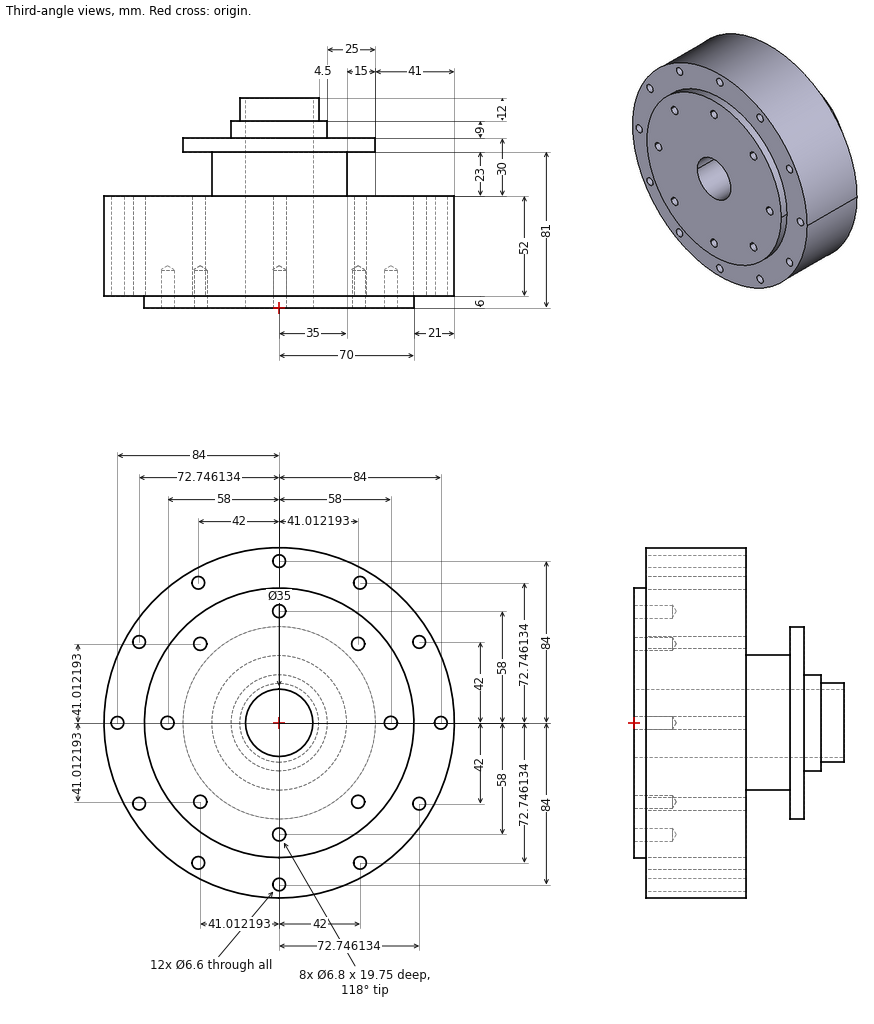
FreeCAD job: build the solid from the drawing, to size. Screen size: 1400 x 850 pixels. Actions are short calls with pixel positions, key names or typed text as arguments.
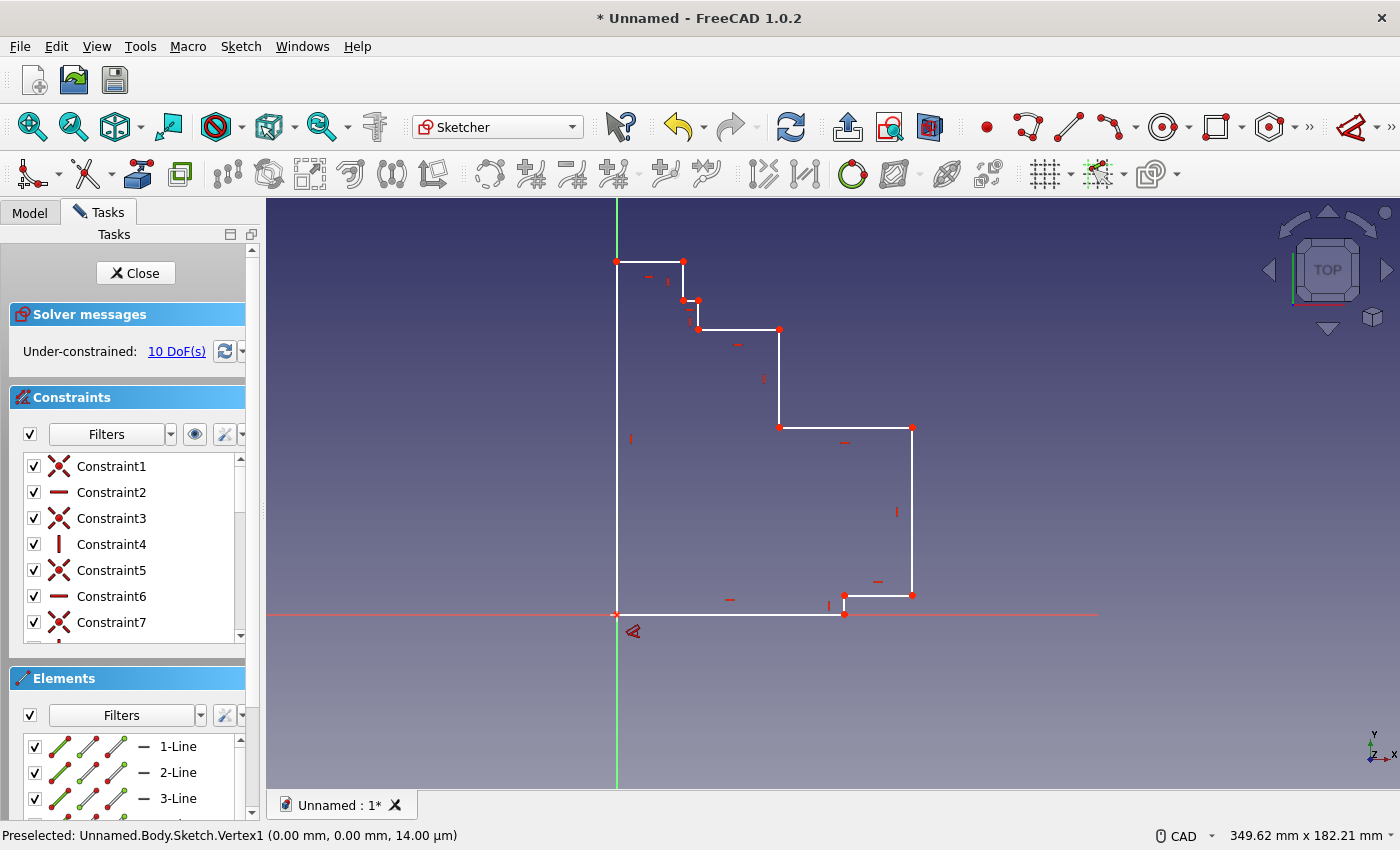
scroll(844, 605, up, 4)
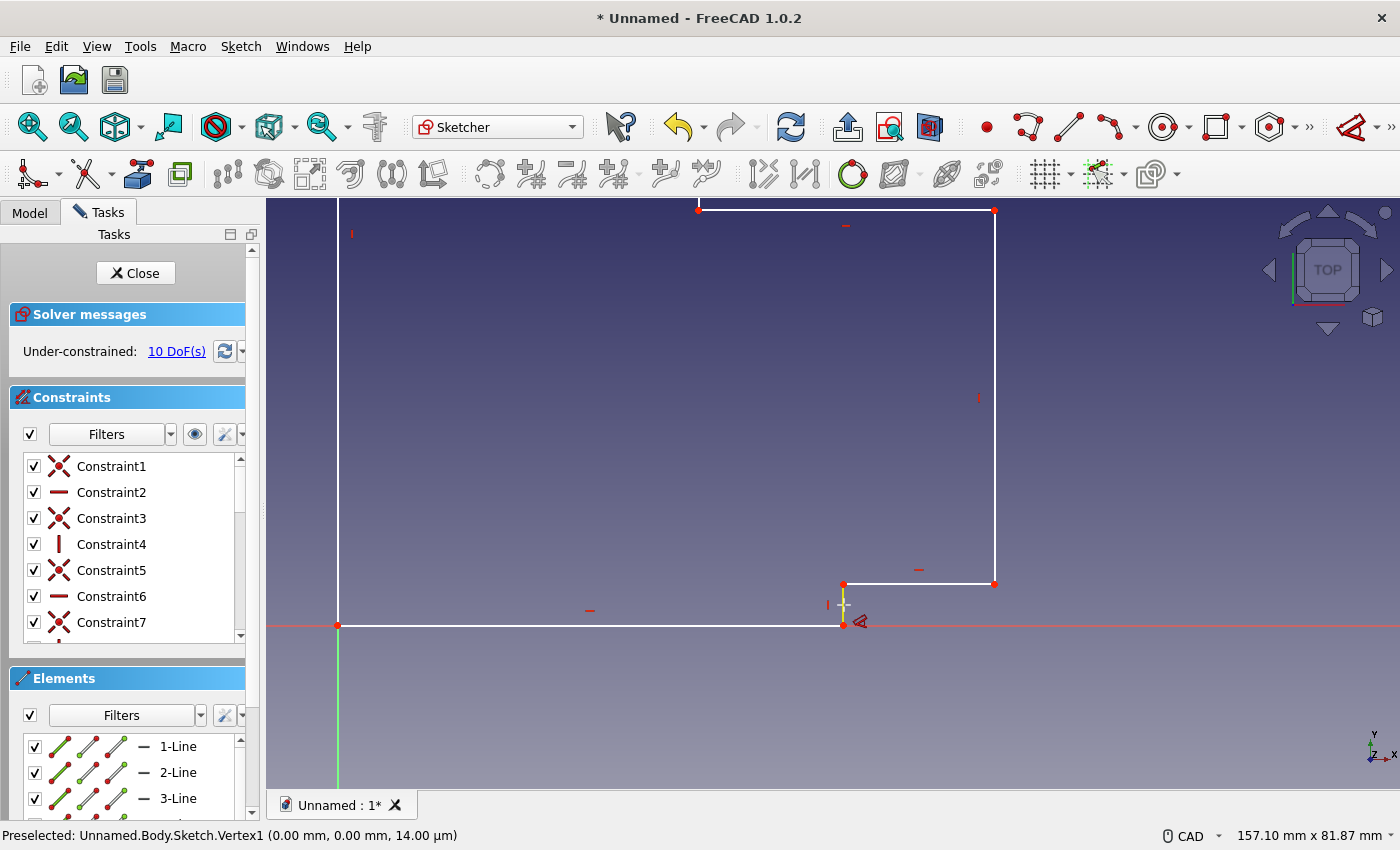
click(843, 605)
click(877, 605)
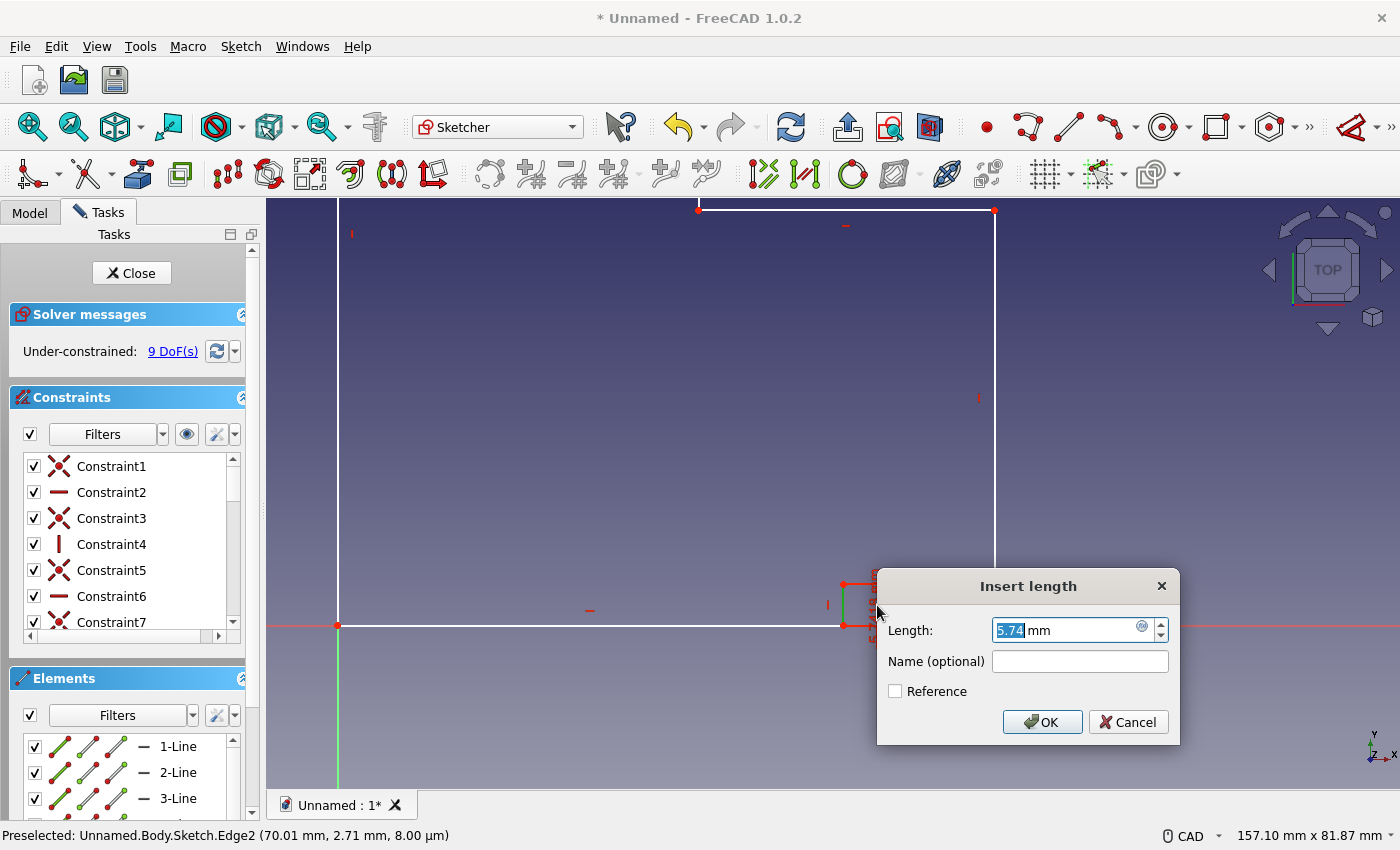
text(6)
key(Return)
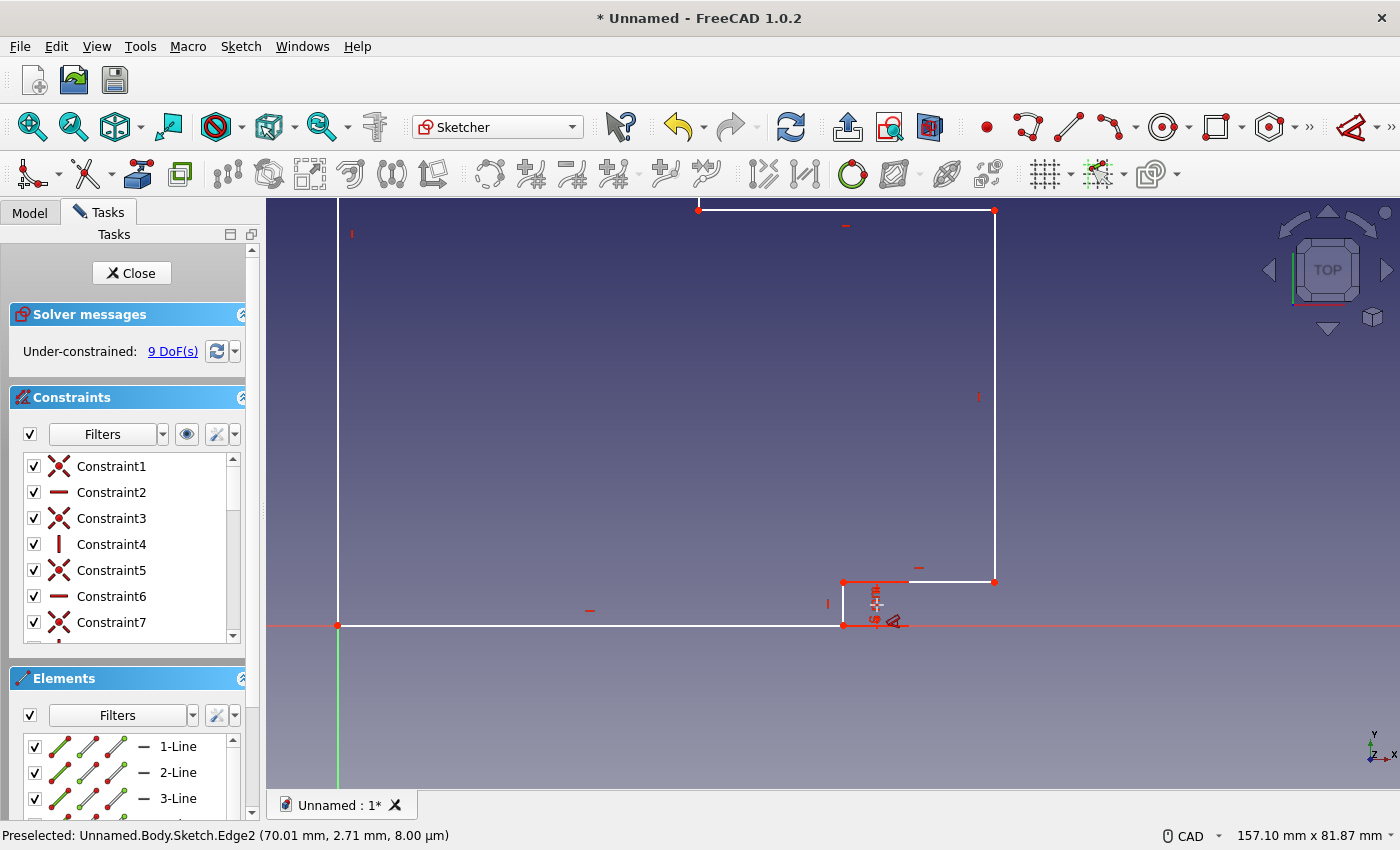
scroll(845, 707, down, 4)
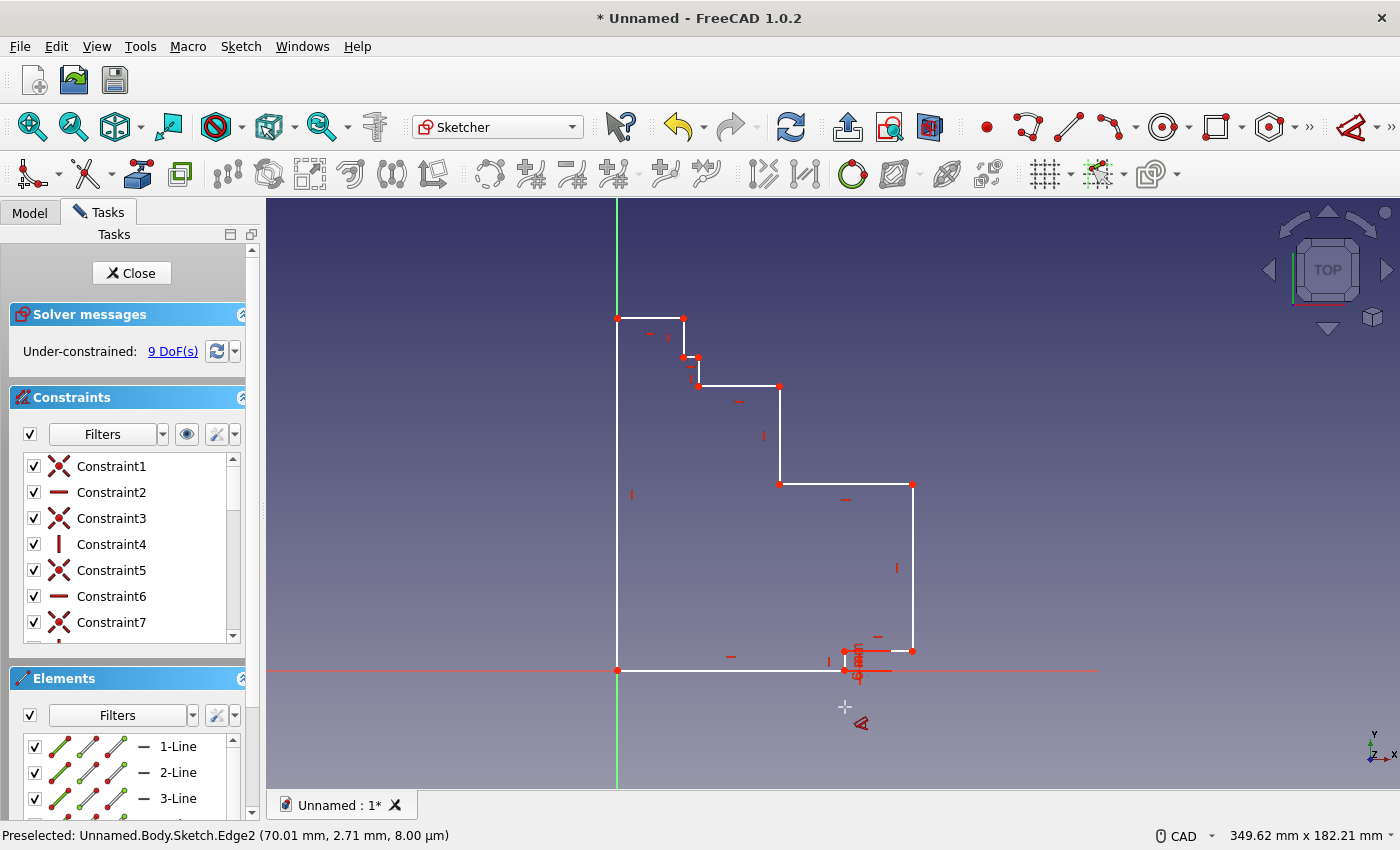
scroll(699, 378, up, 3)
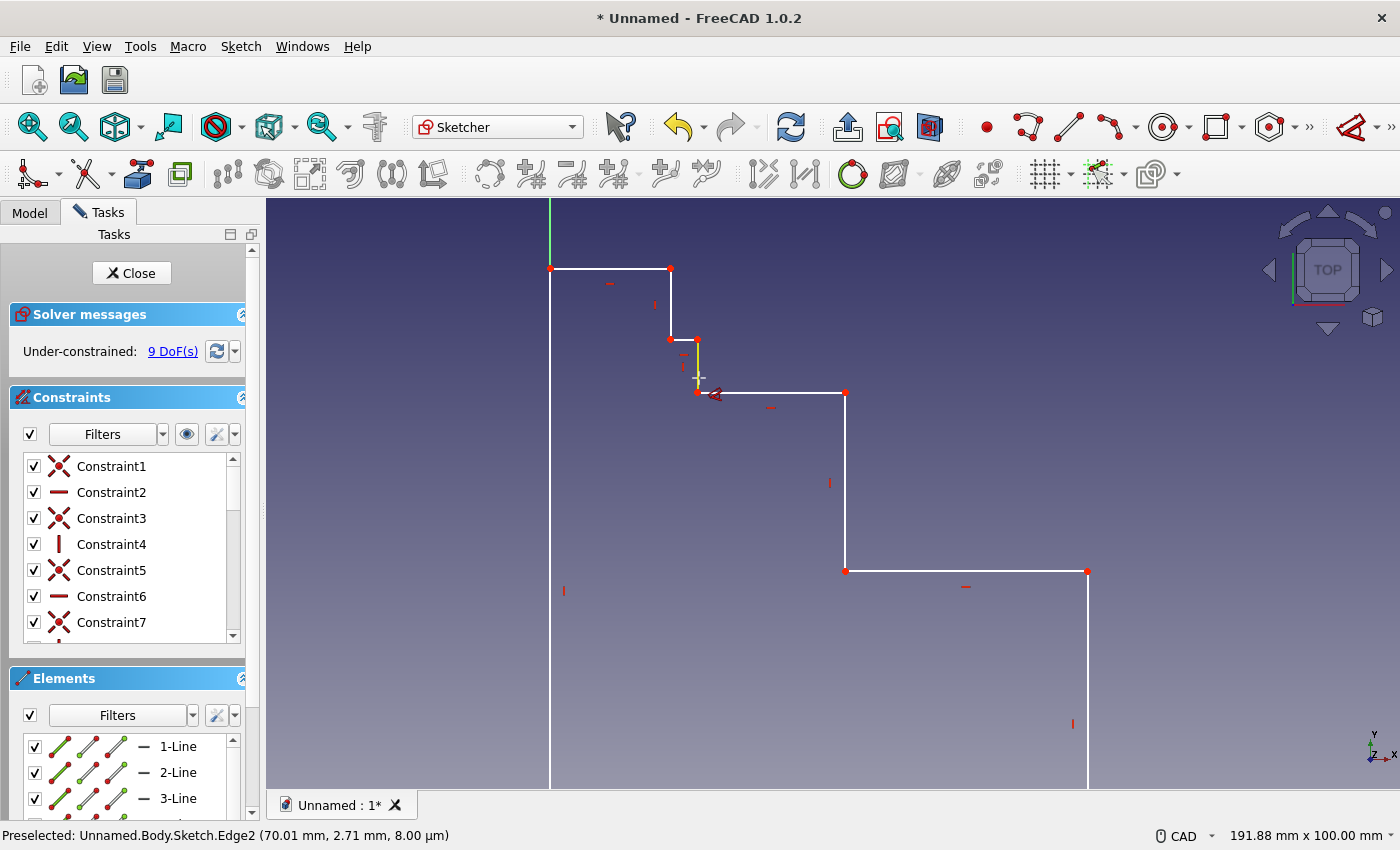
click(698, 377)
click(664, 366)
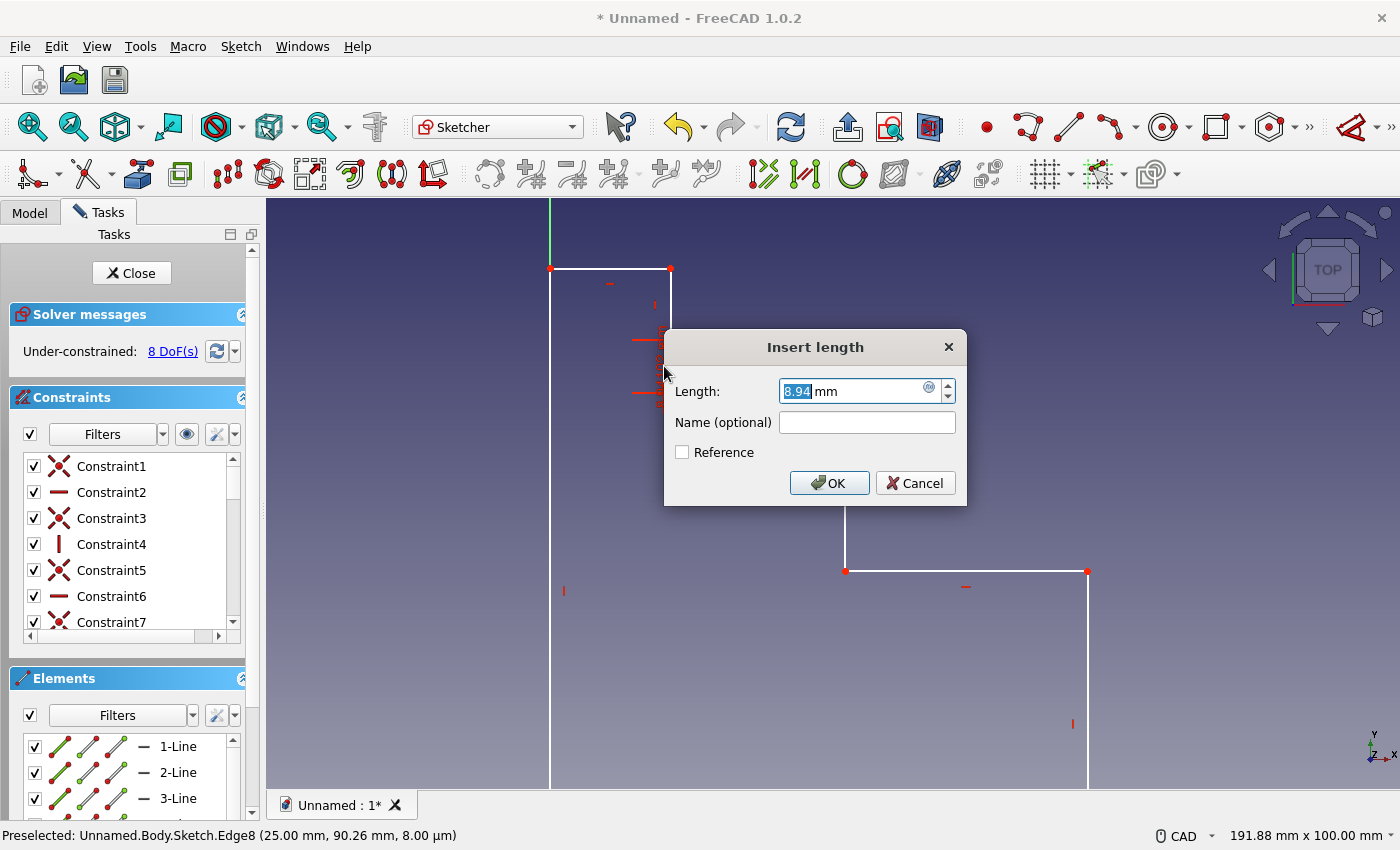
text(9)
key(Return)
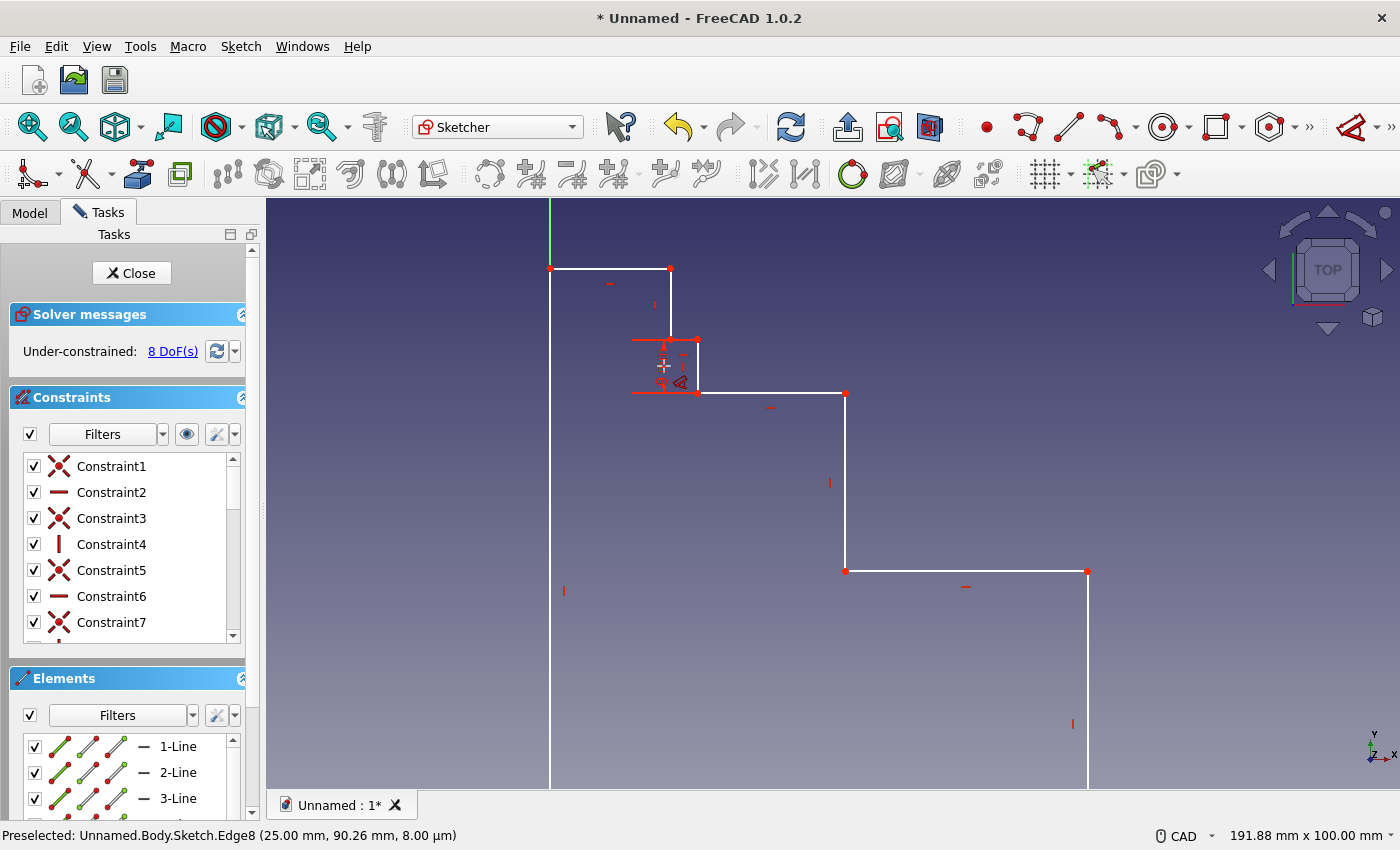
scroll(698, 377, down, 3)